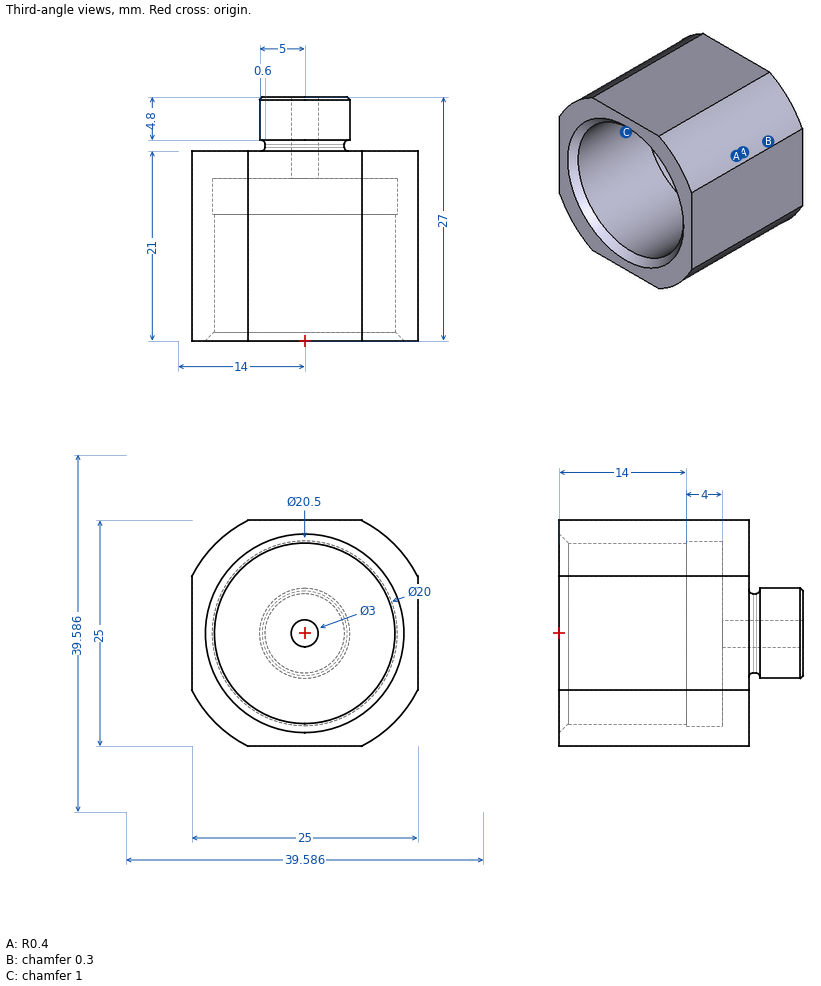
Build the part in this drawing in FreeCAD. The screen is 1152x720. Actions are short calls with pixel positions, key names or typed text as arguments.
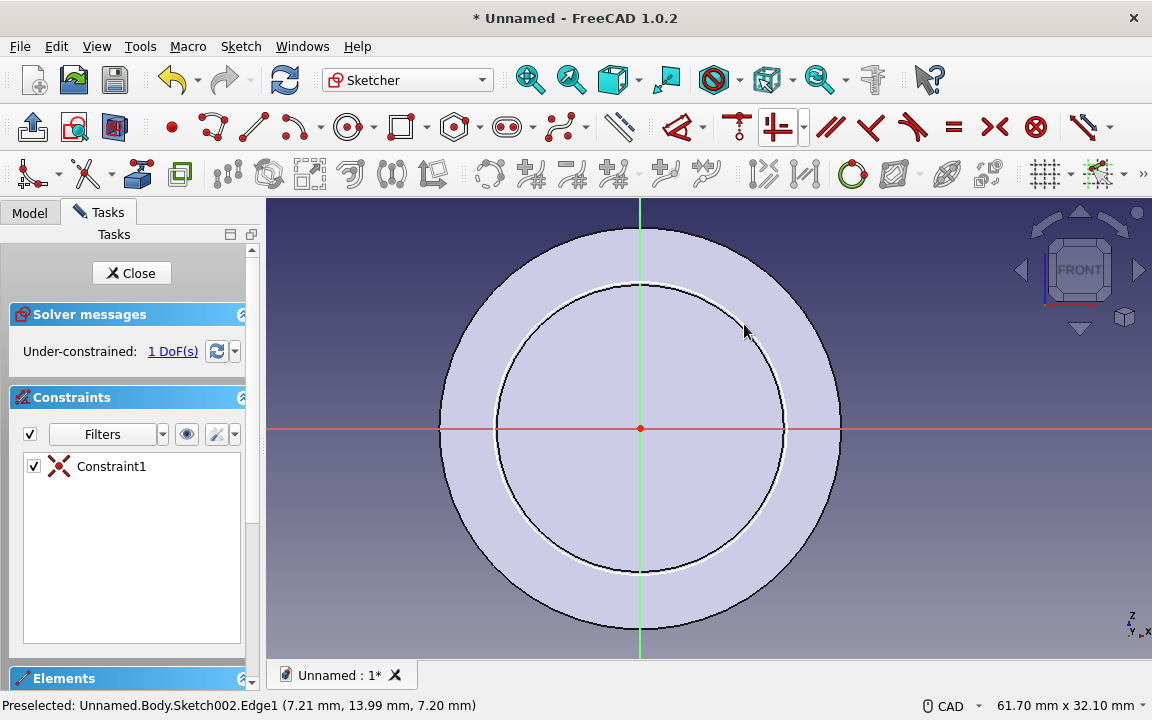
click(676, 128)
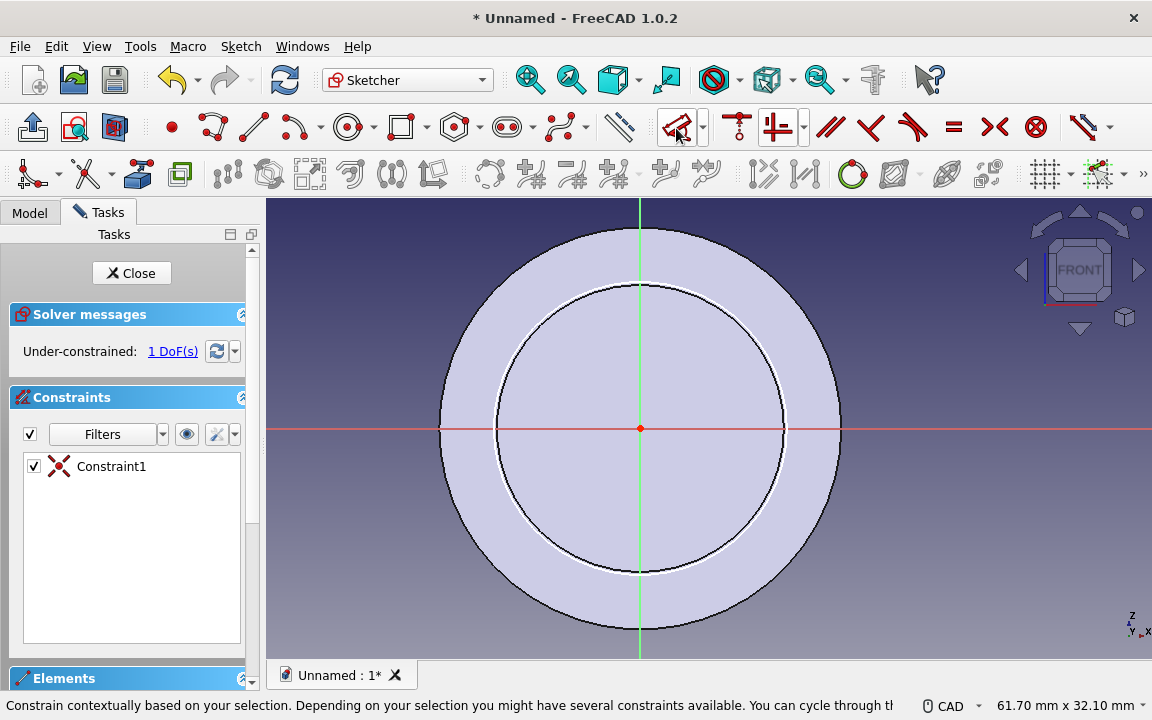
click(744, 325)
click(767, 302)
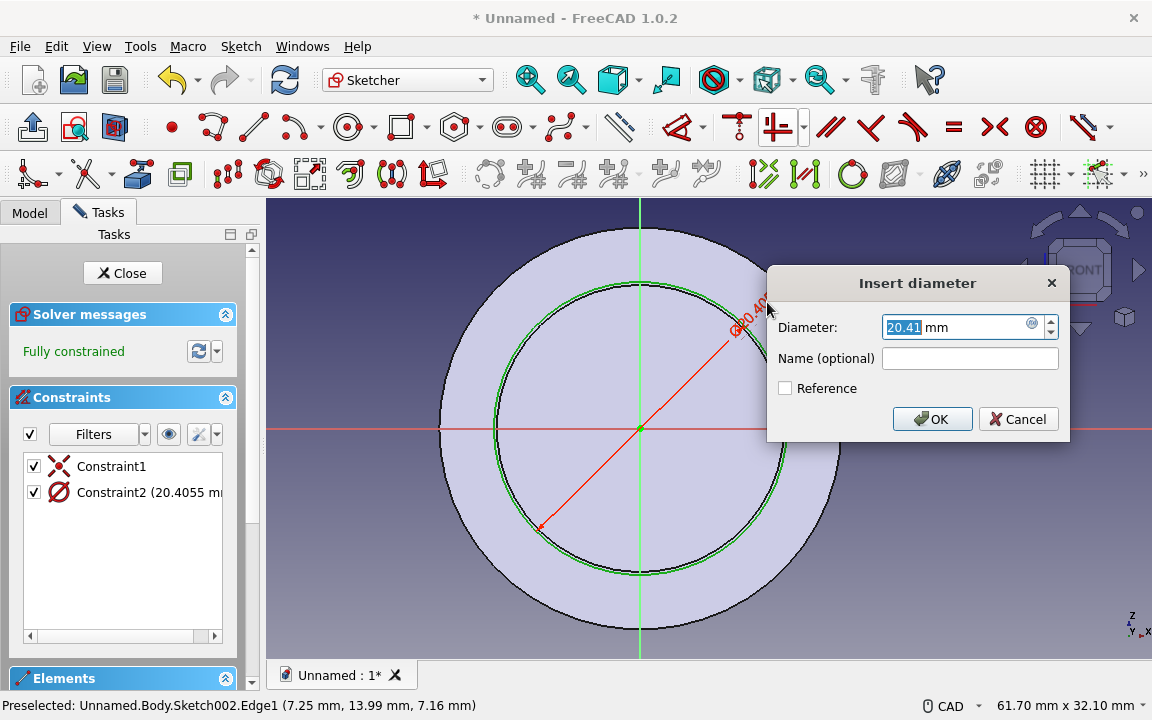
text(20.5)
key(Return)
key(Escape)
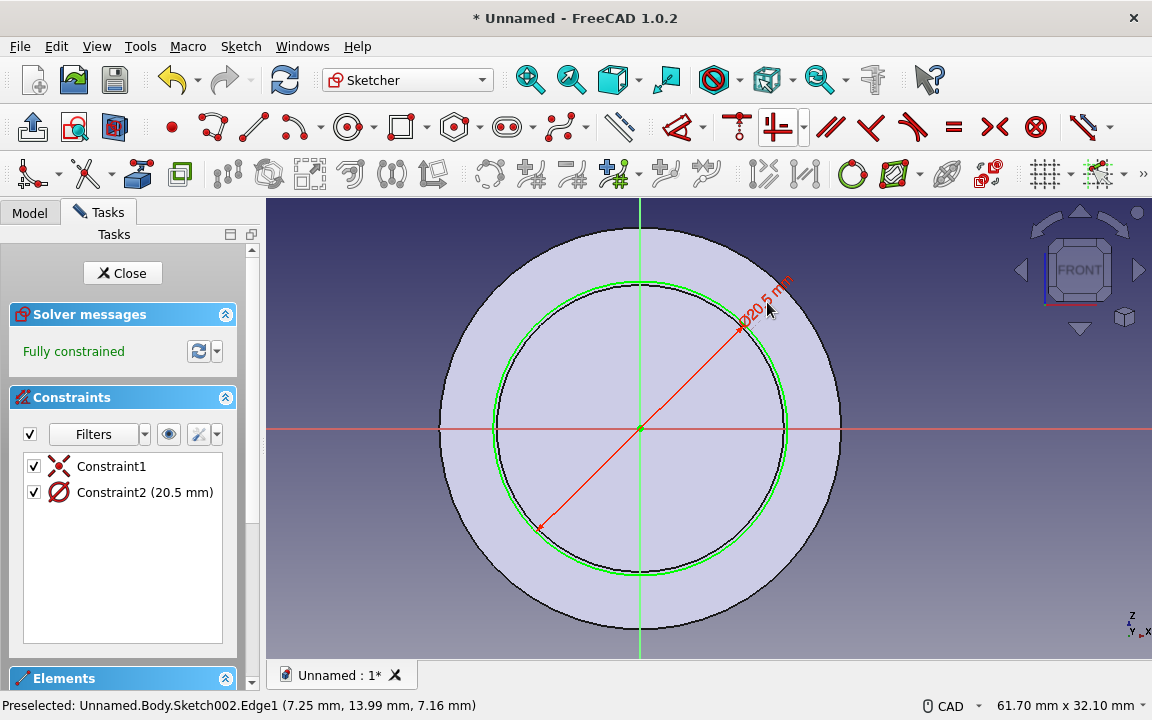
click(123, 273)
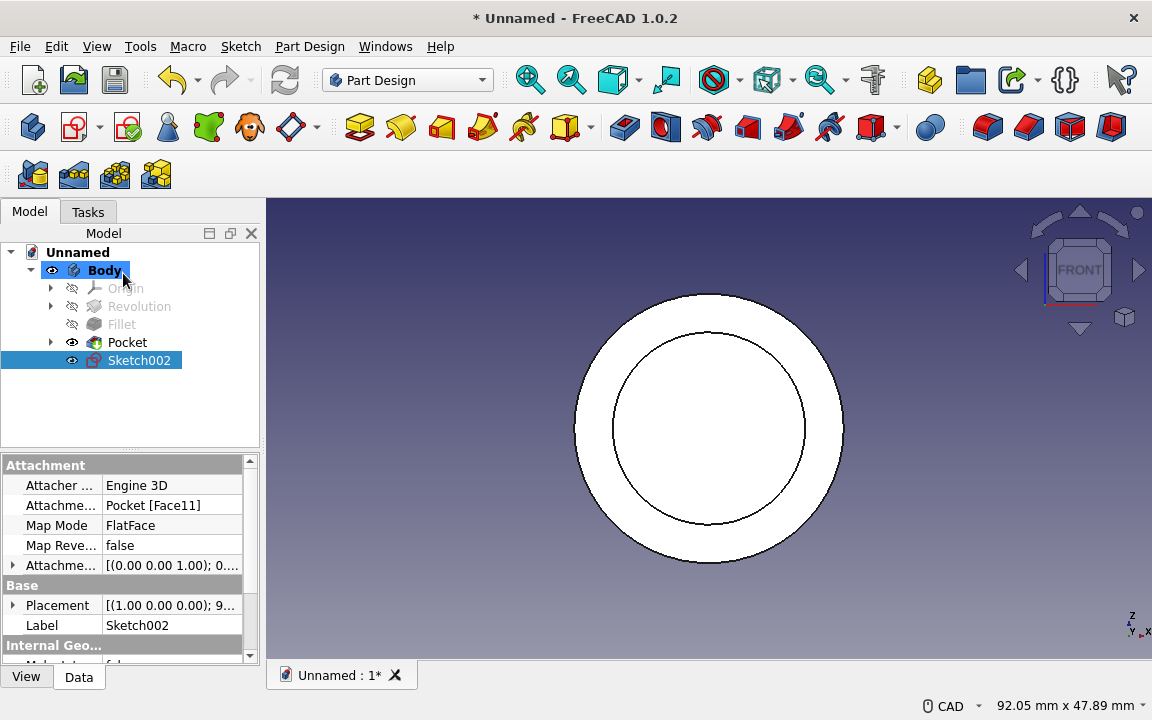
click(625, 128)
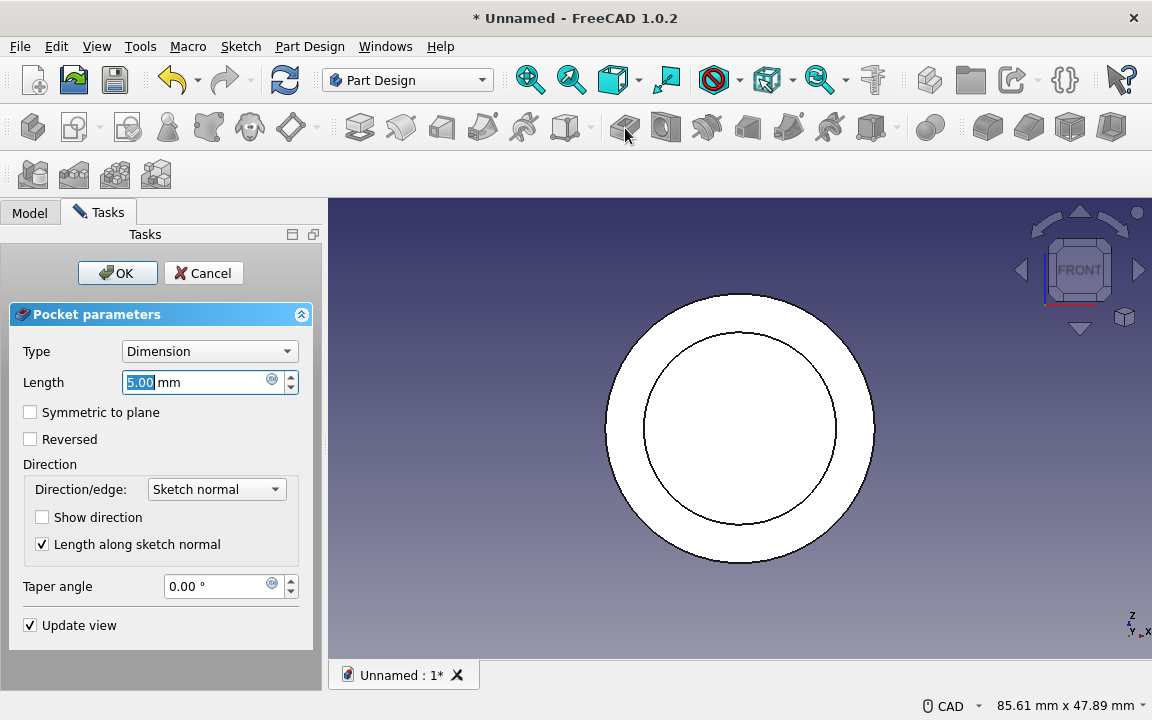
text(4)
key(Tab)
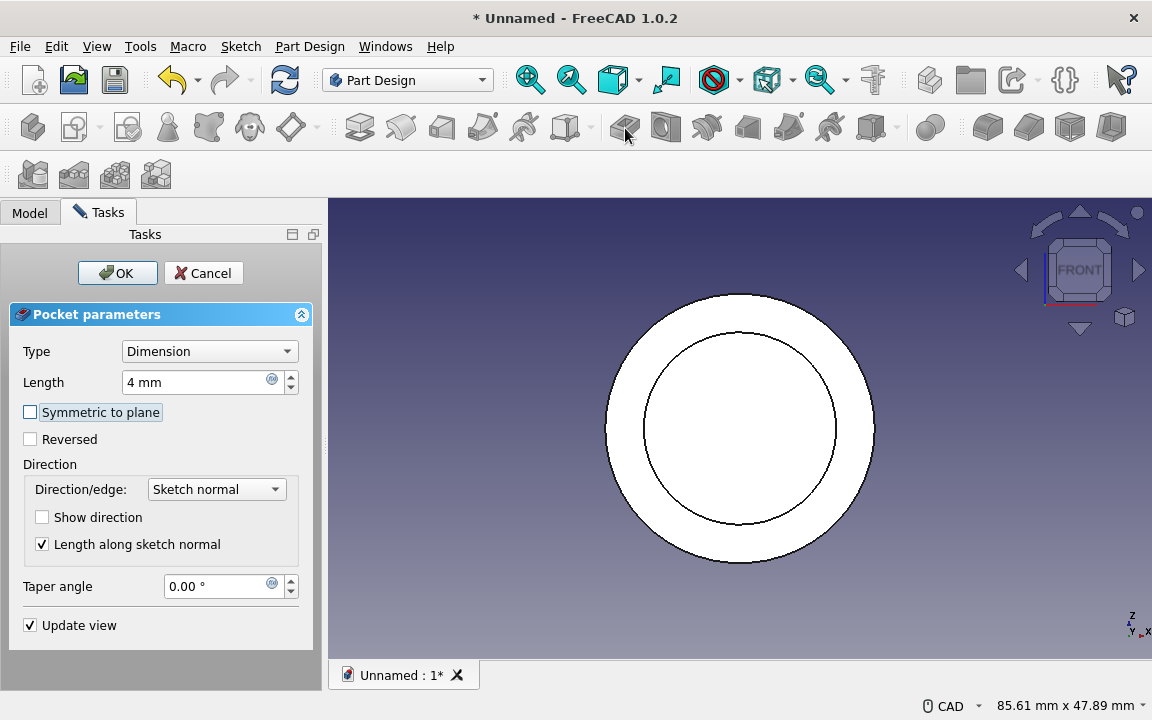
click(118, 273)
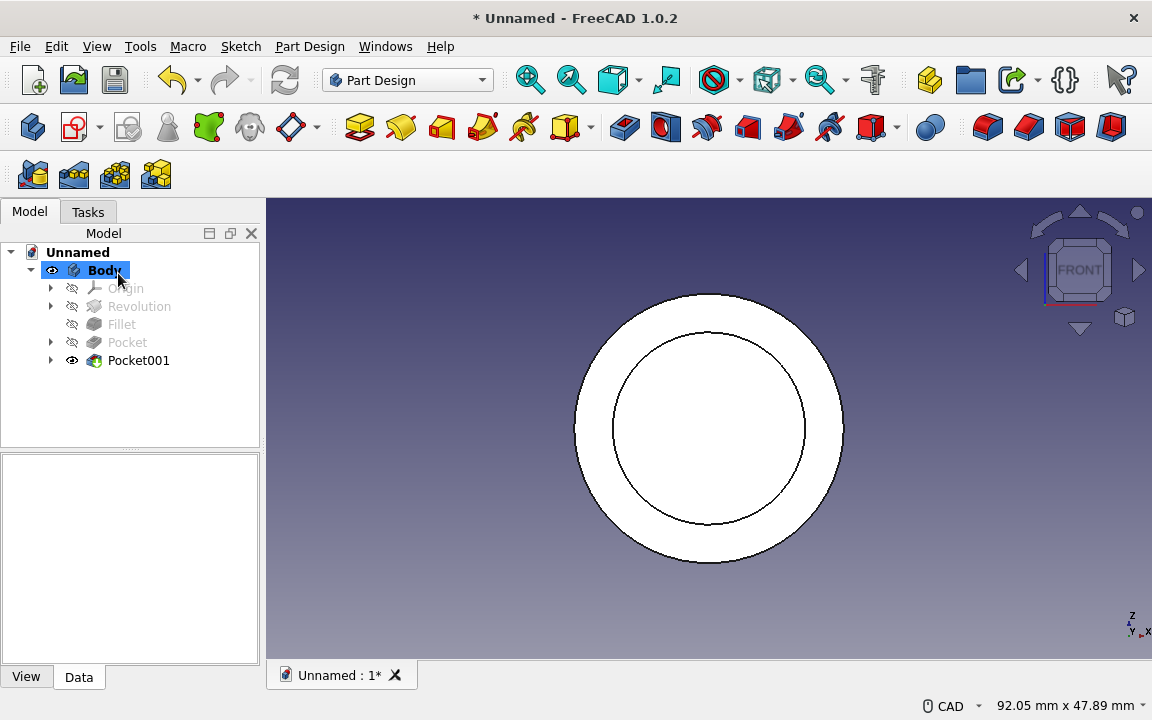
click(709, 427)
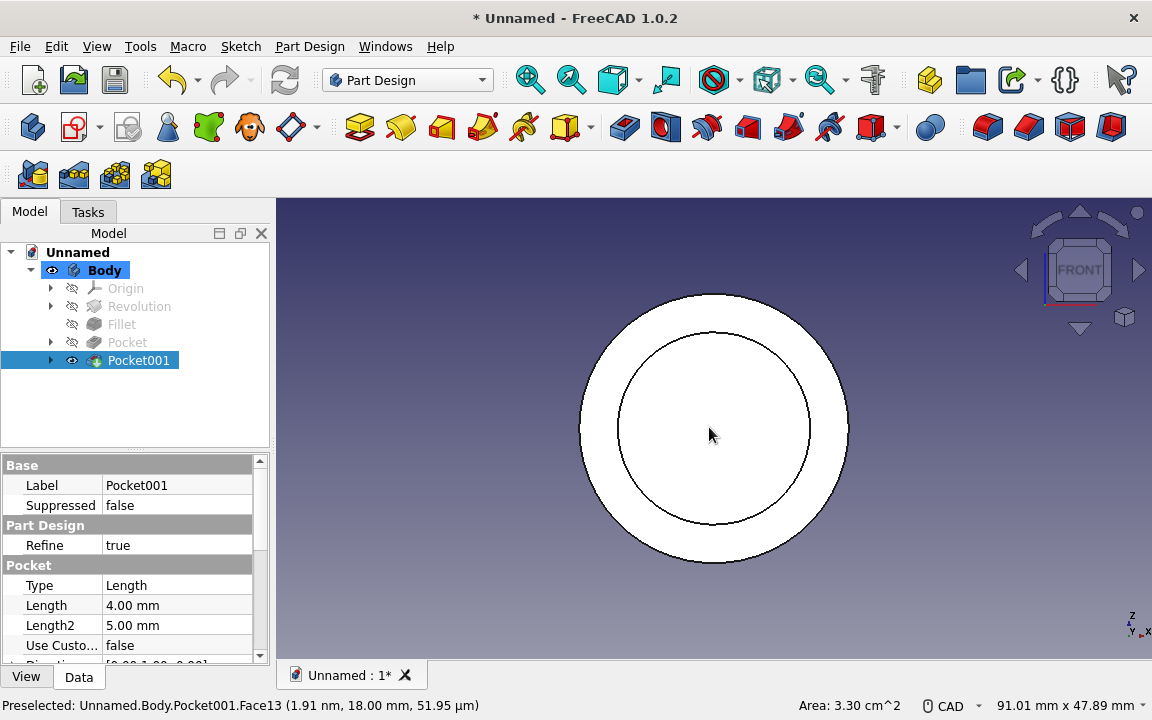
click(74, 128)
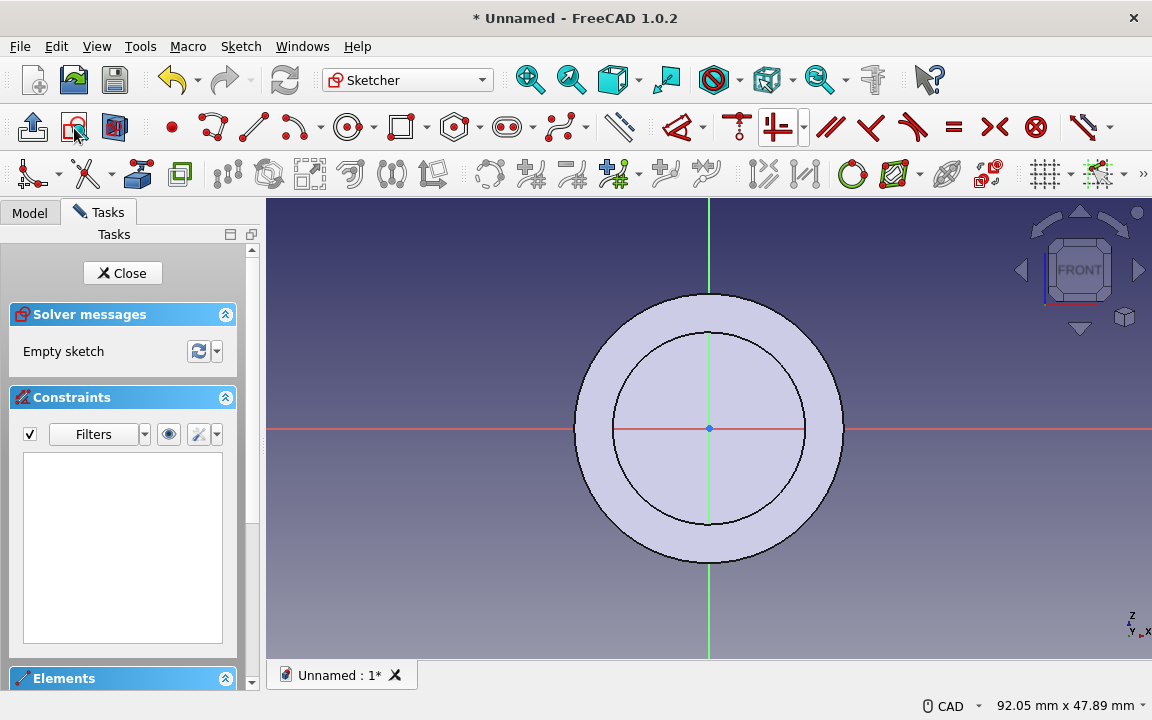
click(115, 128)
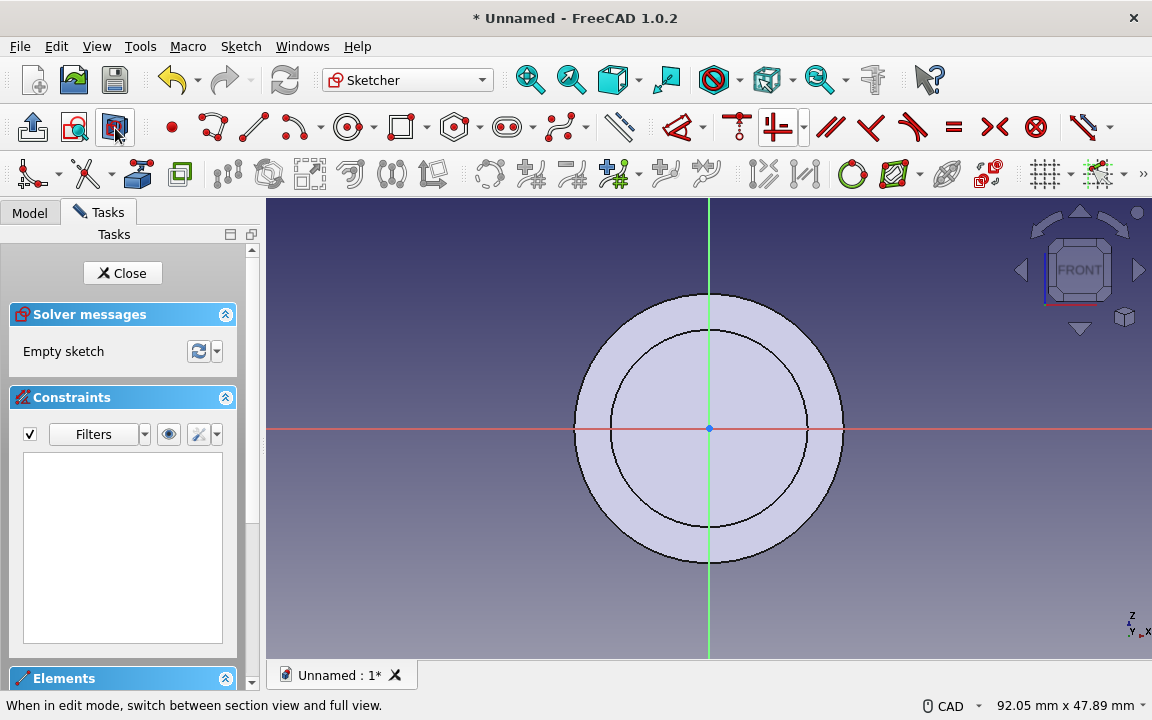
scroll(718, 428, up, 11)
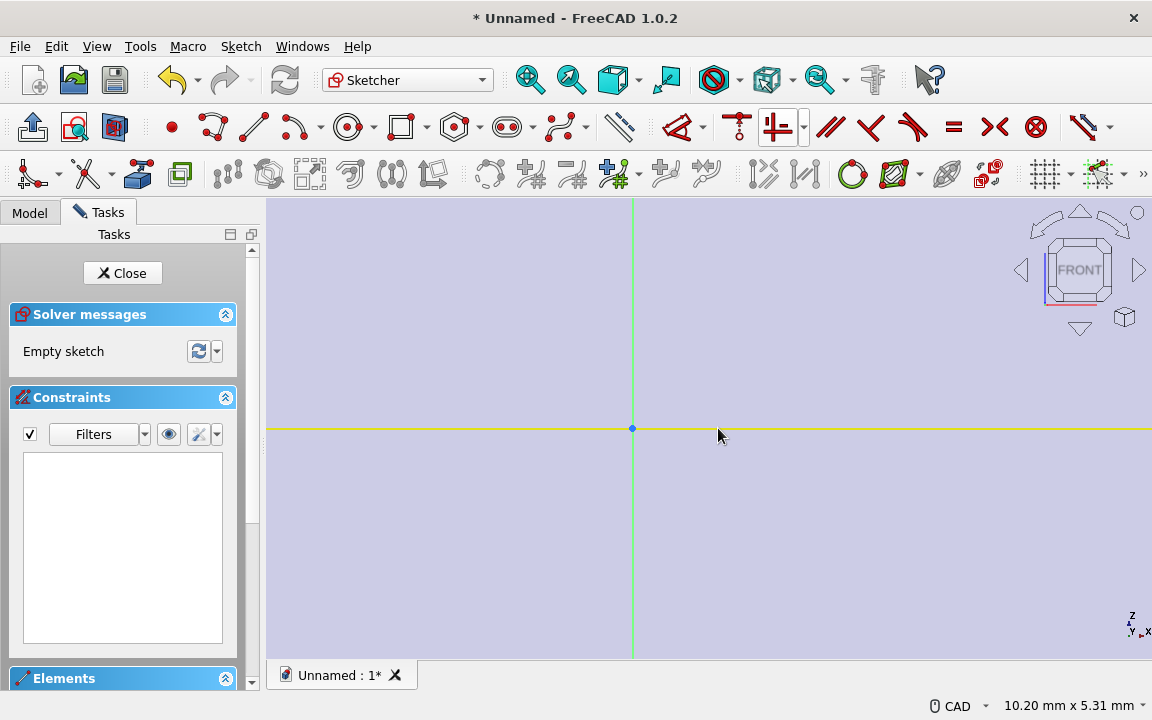
click(348, 128)